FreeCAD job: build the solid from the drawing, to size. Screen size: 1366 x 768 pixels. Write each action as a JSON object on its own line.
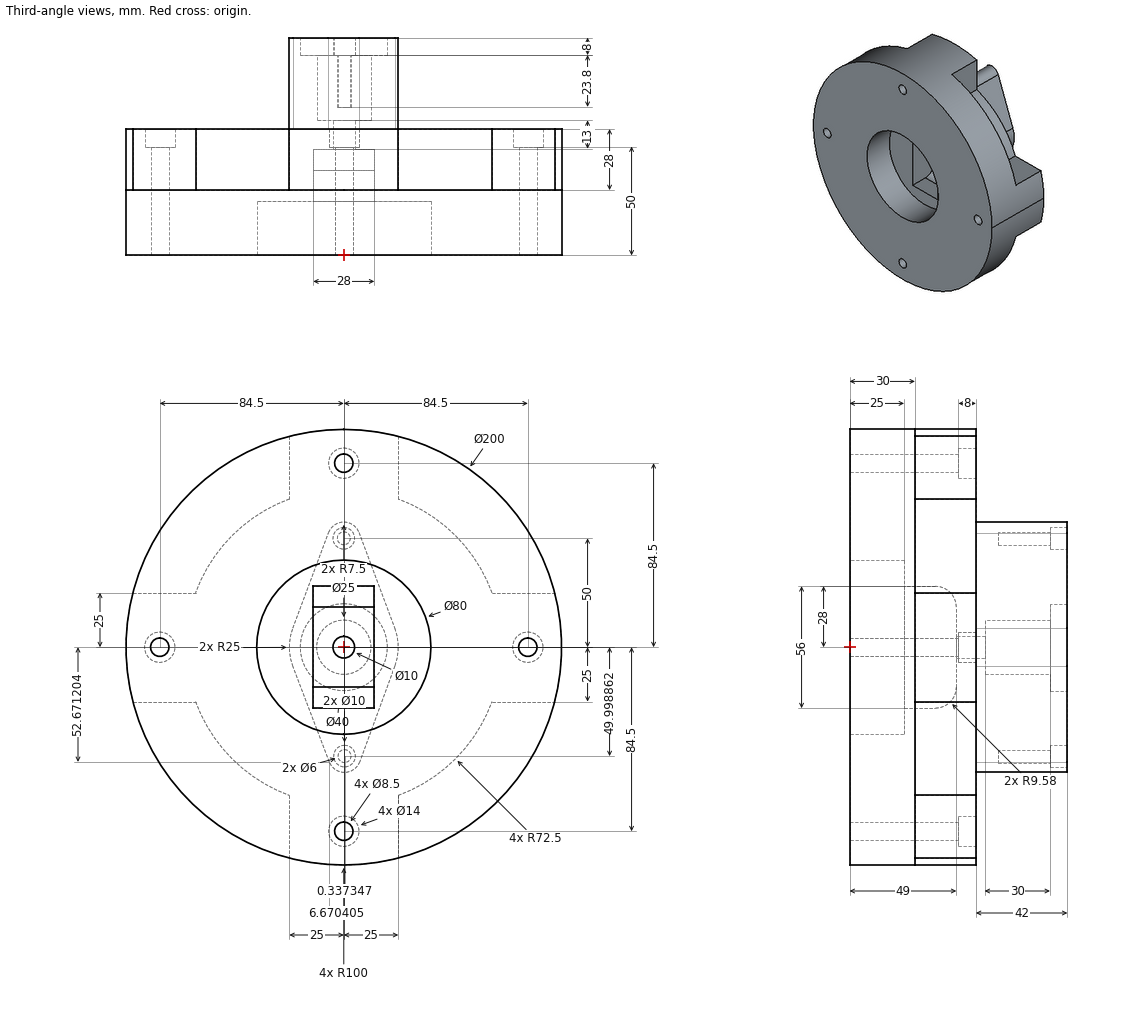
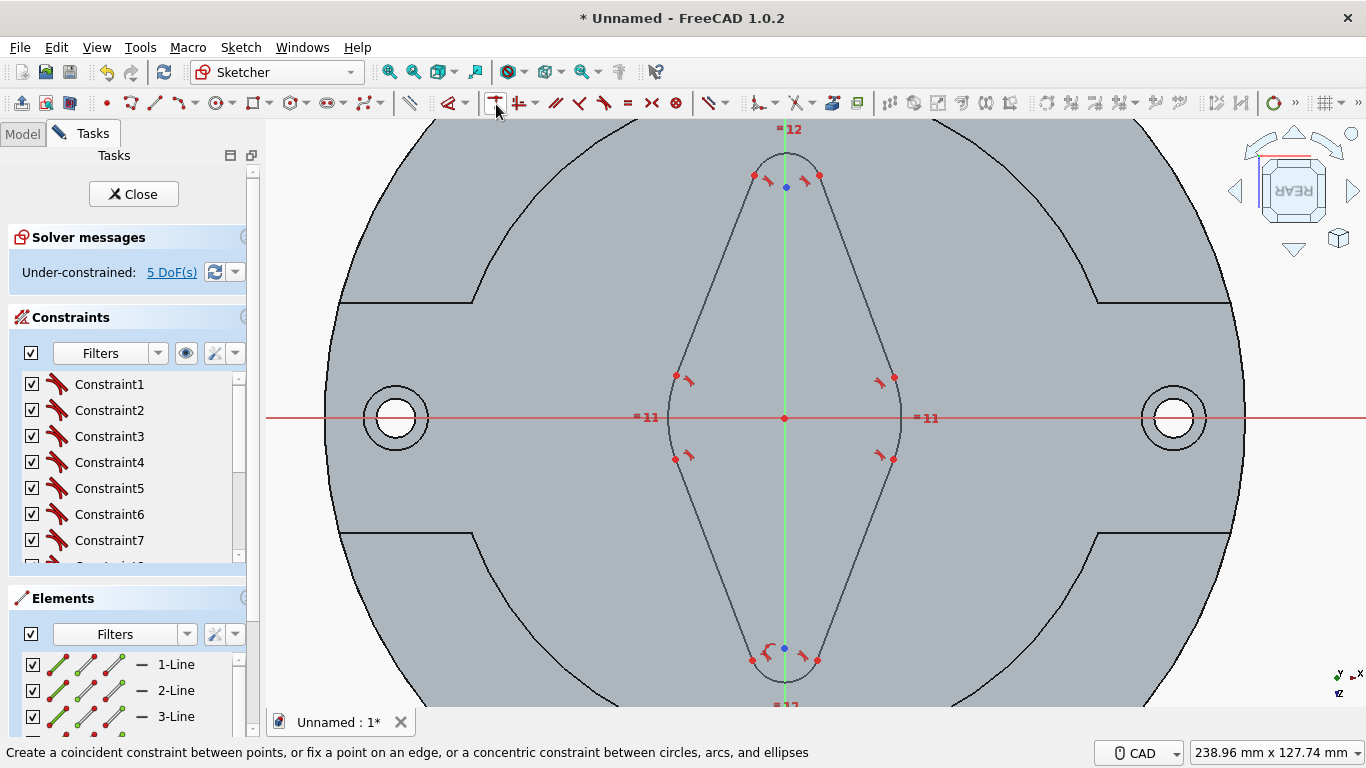
{"action": "left_click", "coordinate": [670, 401]}
{"action": "left_click", "coordinate": [638, 396]}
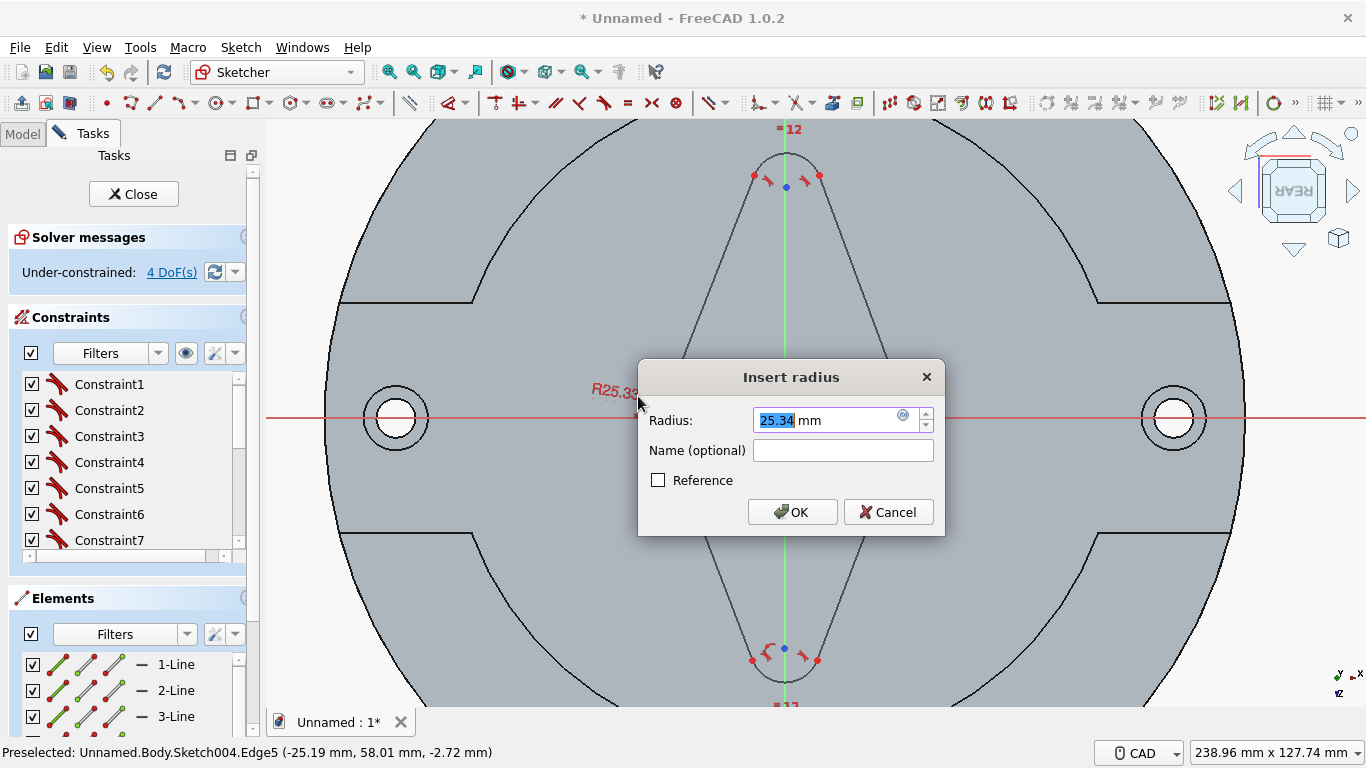
{"action": "type", "text": "25"}
{"action": "key", "text": "Return"}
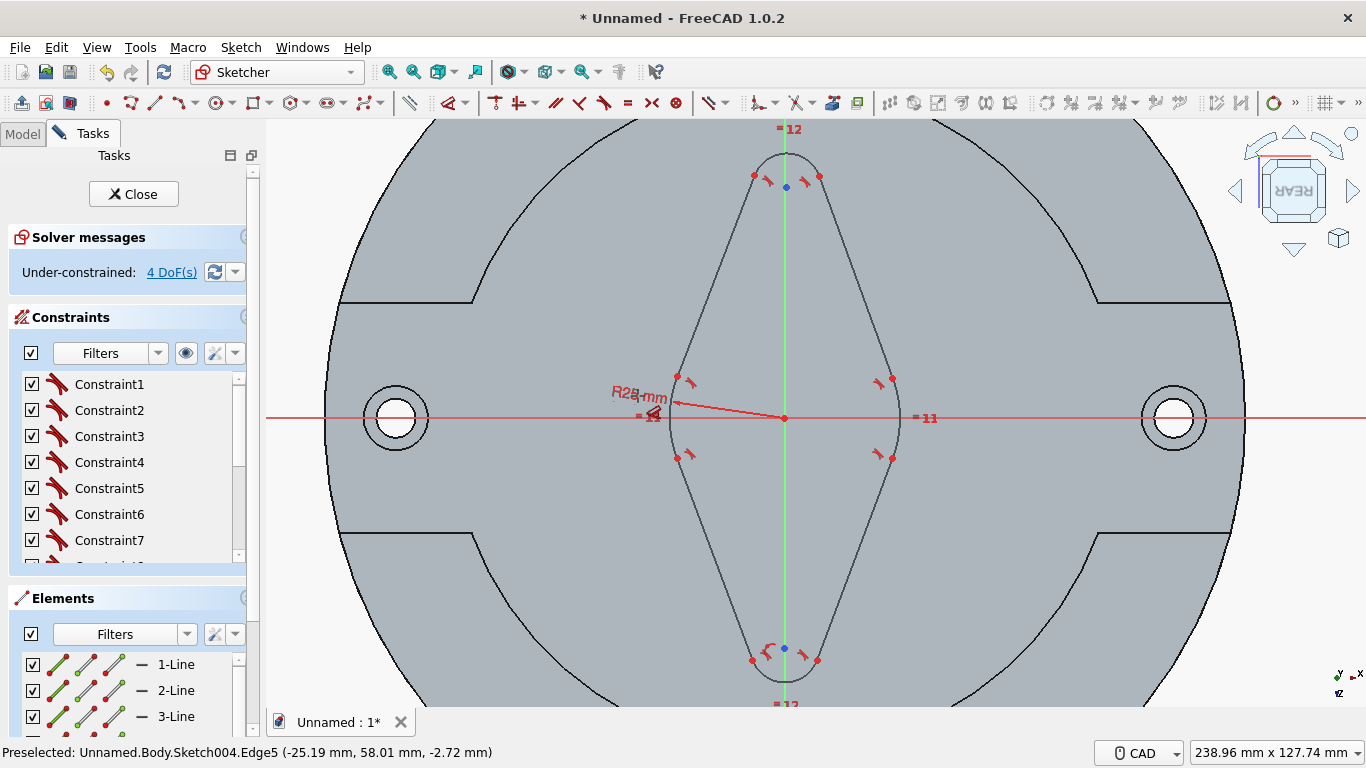
{"action": "left_click", "coordinate": [769, 678]}
{"action": "left_click", "coordinate": [719, 654]}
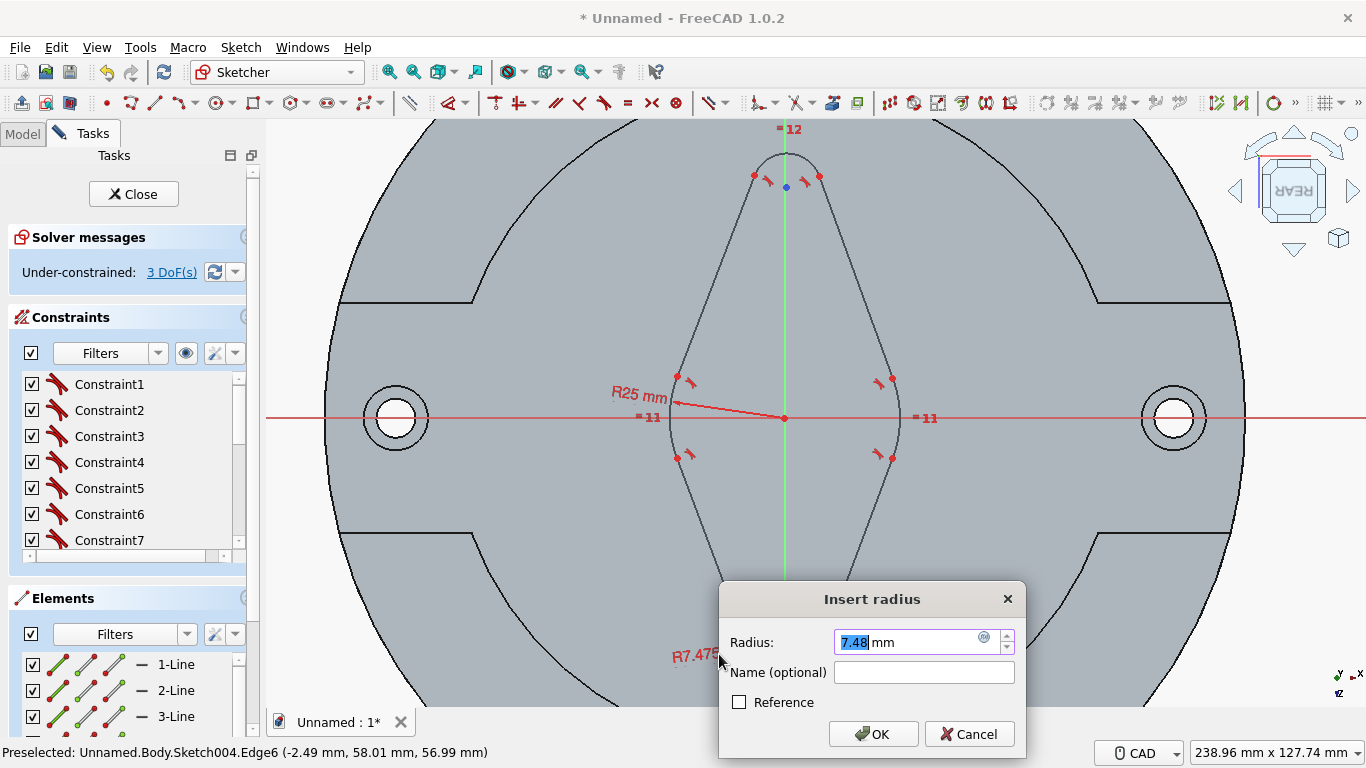
{"action": "type", "text": "7.5"}
{"action": "key", "text": "Return"}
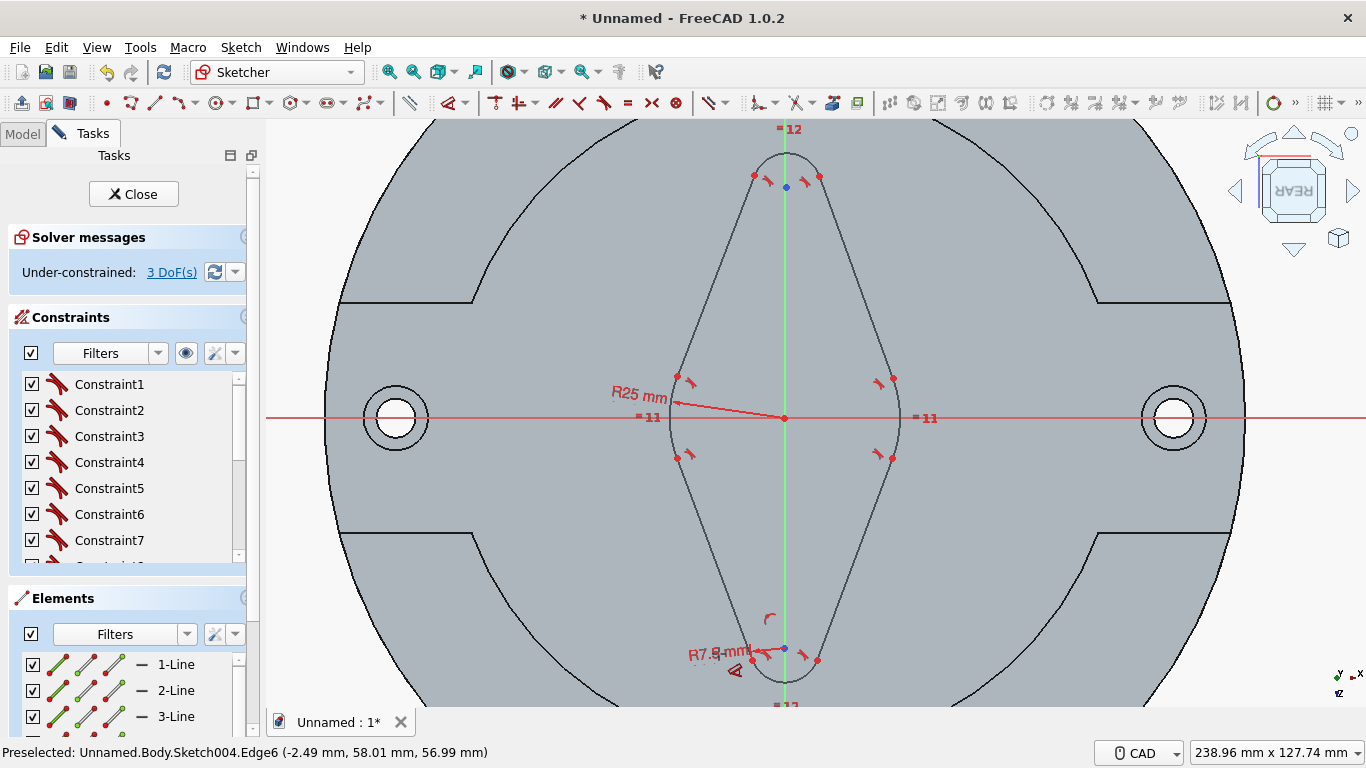
{"action": "left_click", "coordinate": [785, 648]}
{"action": "left_click", "coordinate": [819, 533]}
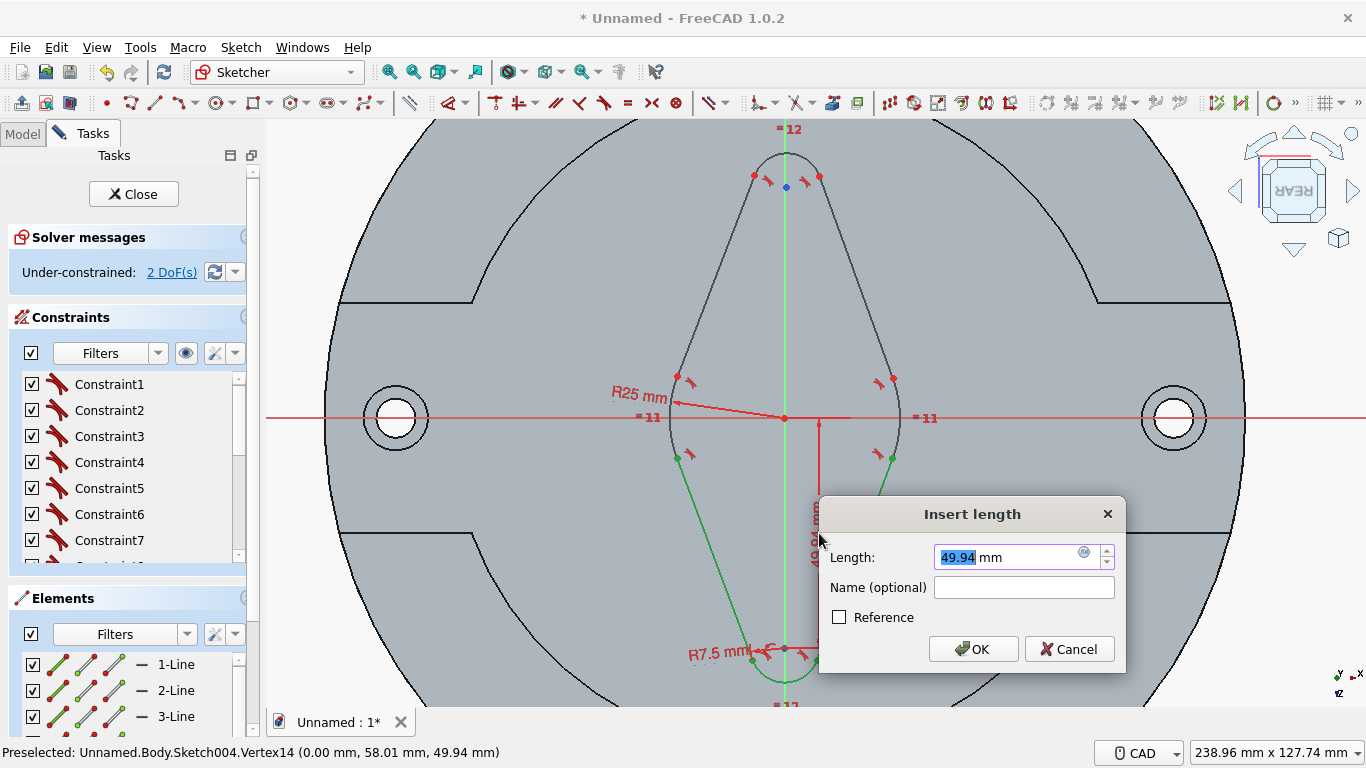
{"action": "type", "text": "50"}
{"action": "key", "text": "Return"}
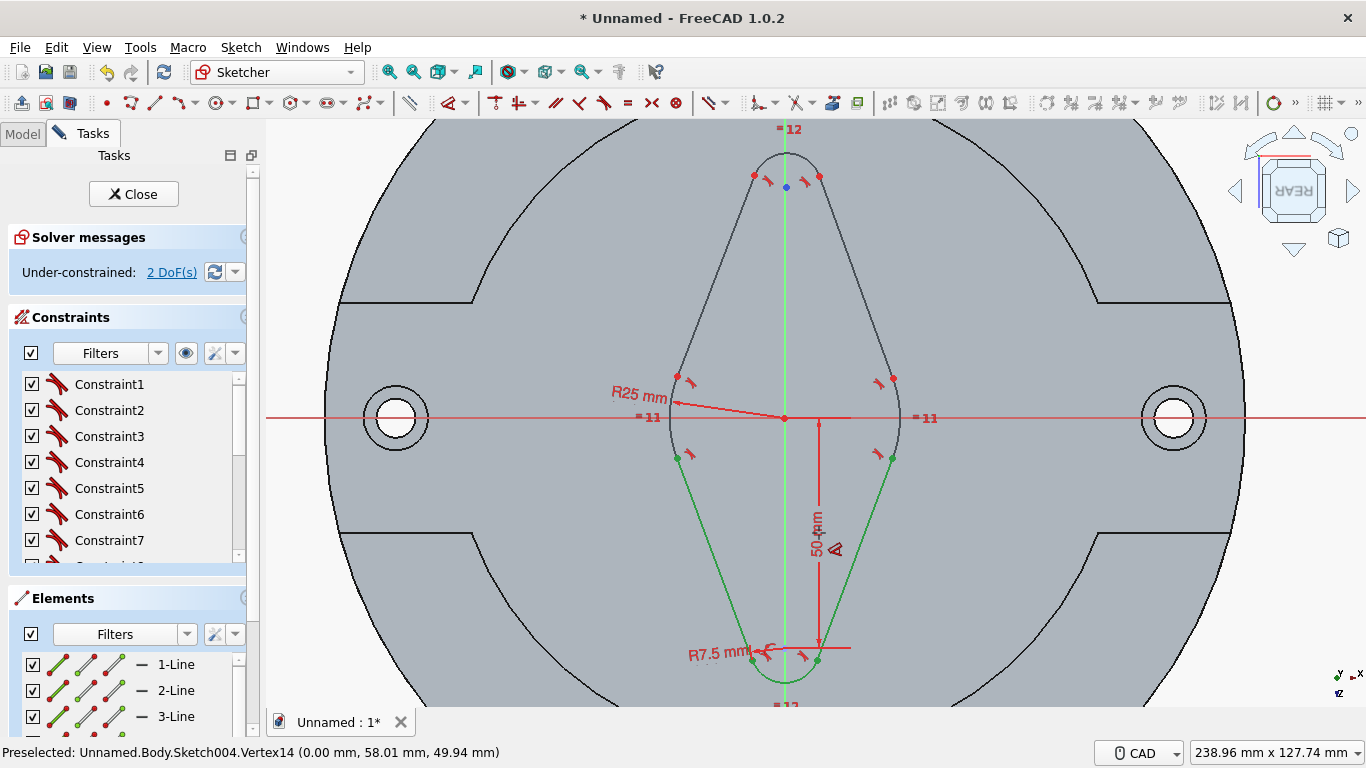
{"action": "scroll", "coordinate": [755, 176], "scroll_direction": "up", "scroll_amount": 2}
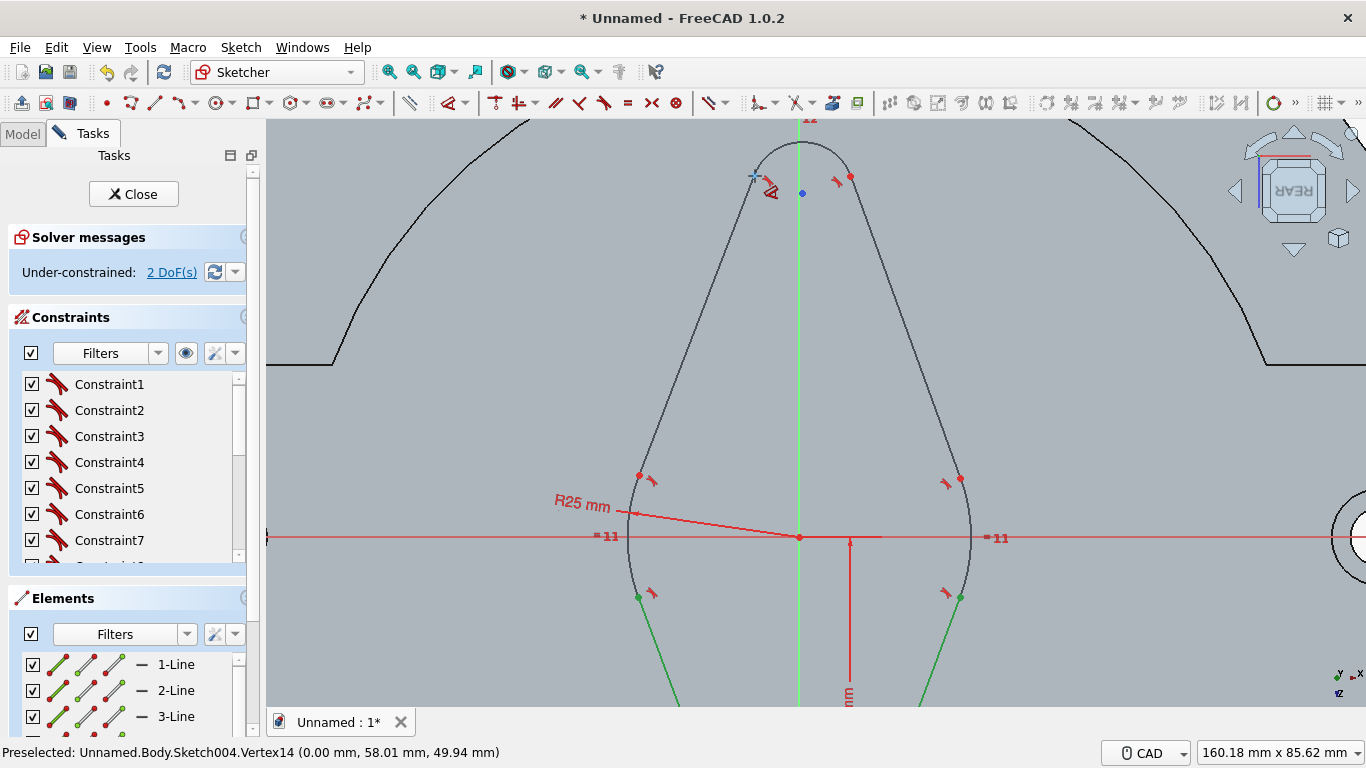
{"action": "left_click", "coordinate": [754, 175]}
{"action": "left_click", "coordinate": [777, 571]}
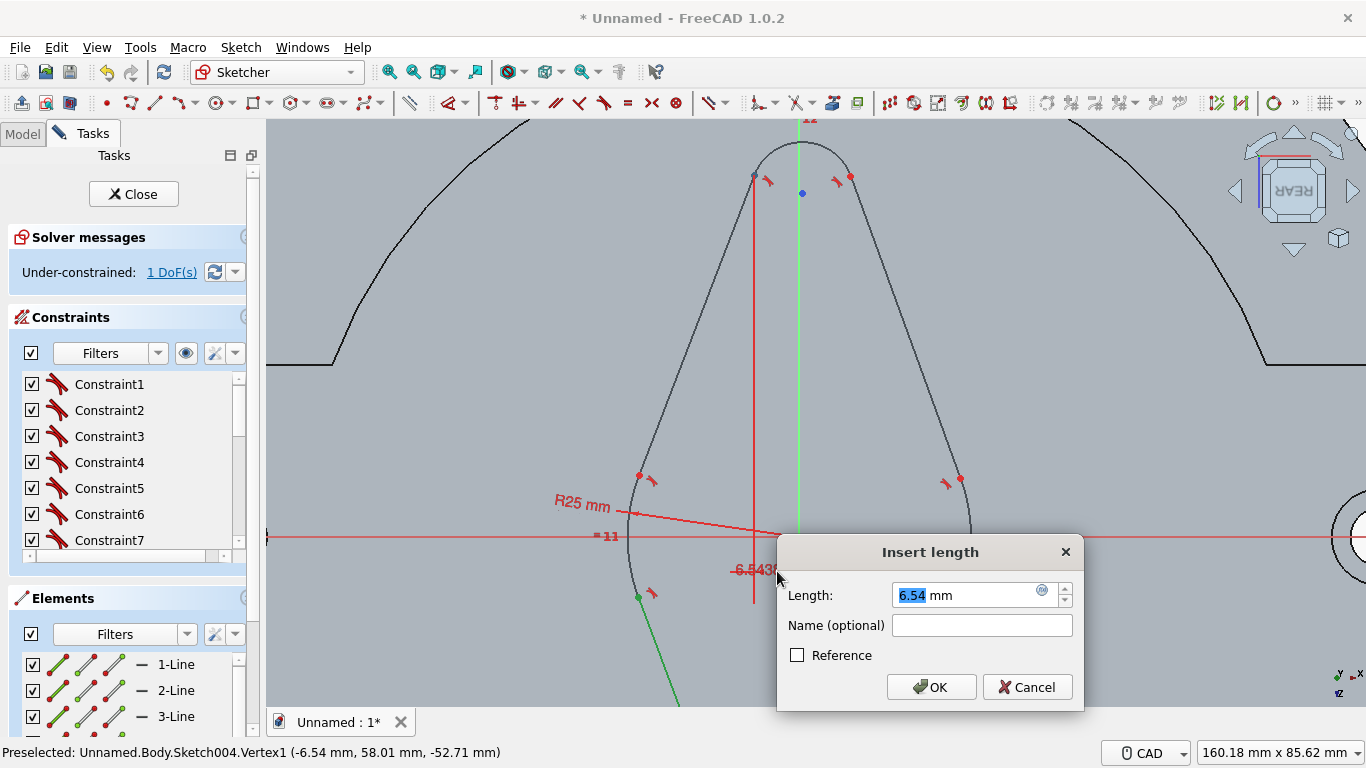
{"action": "type", "text": "6.670405"}
{"action": "key", "text": "Return"}